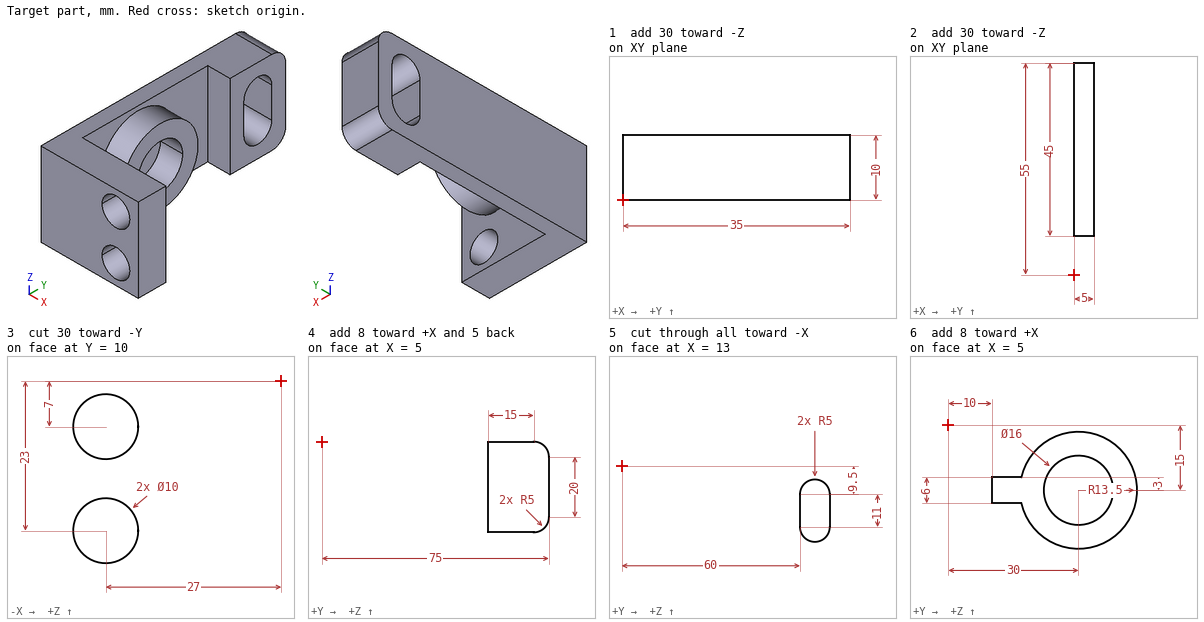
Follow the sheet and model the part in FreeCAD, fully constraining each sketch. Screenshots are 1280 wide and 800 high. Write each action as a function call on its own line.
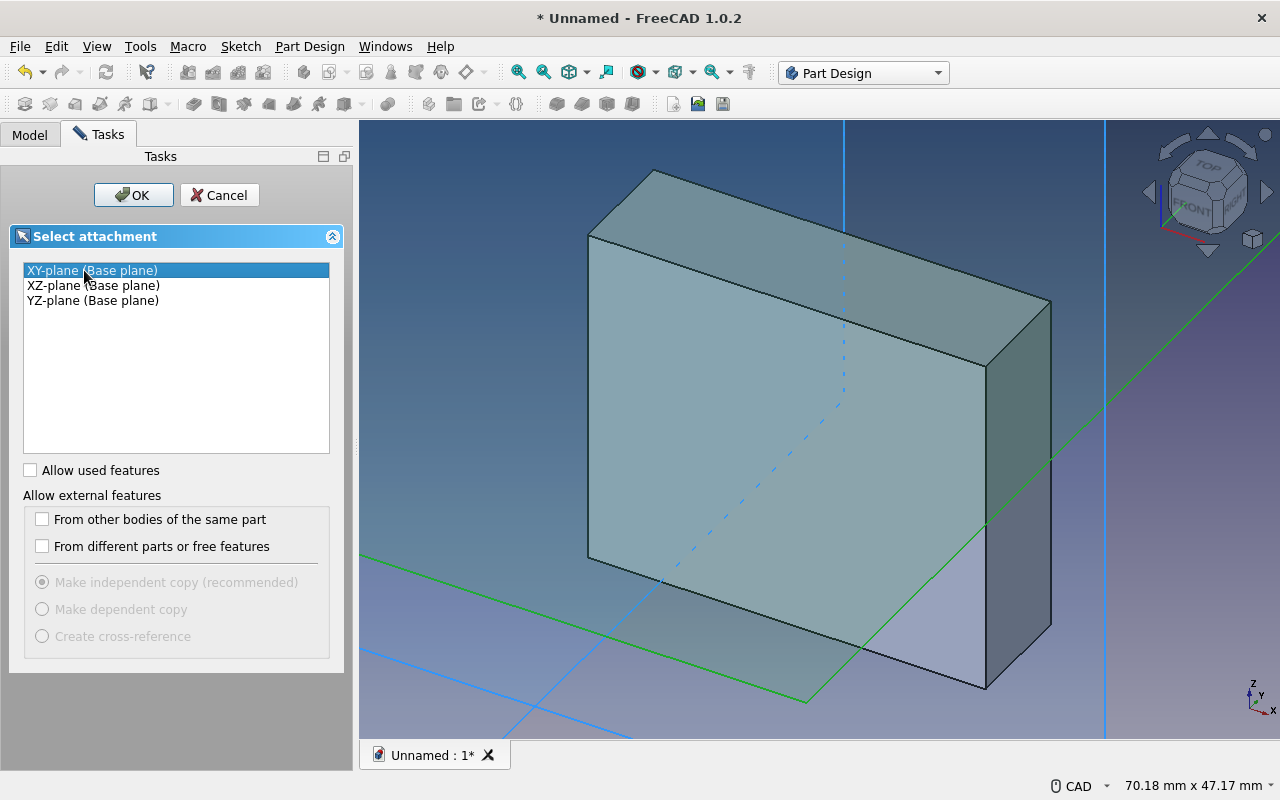
click(134, 195)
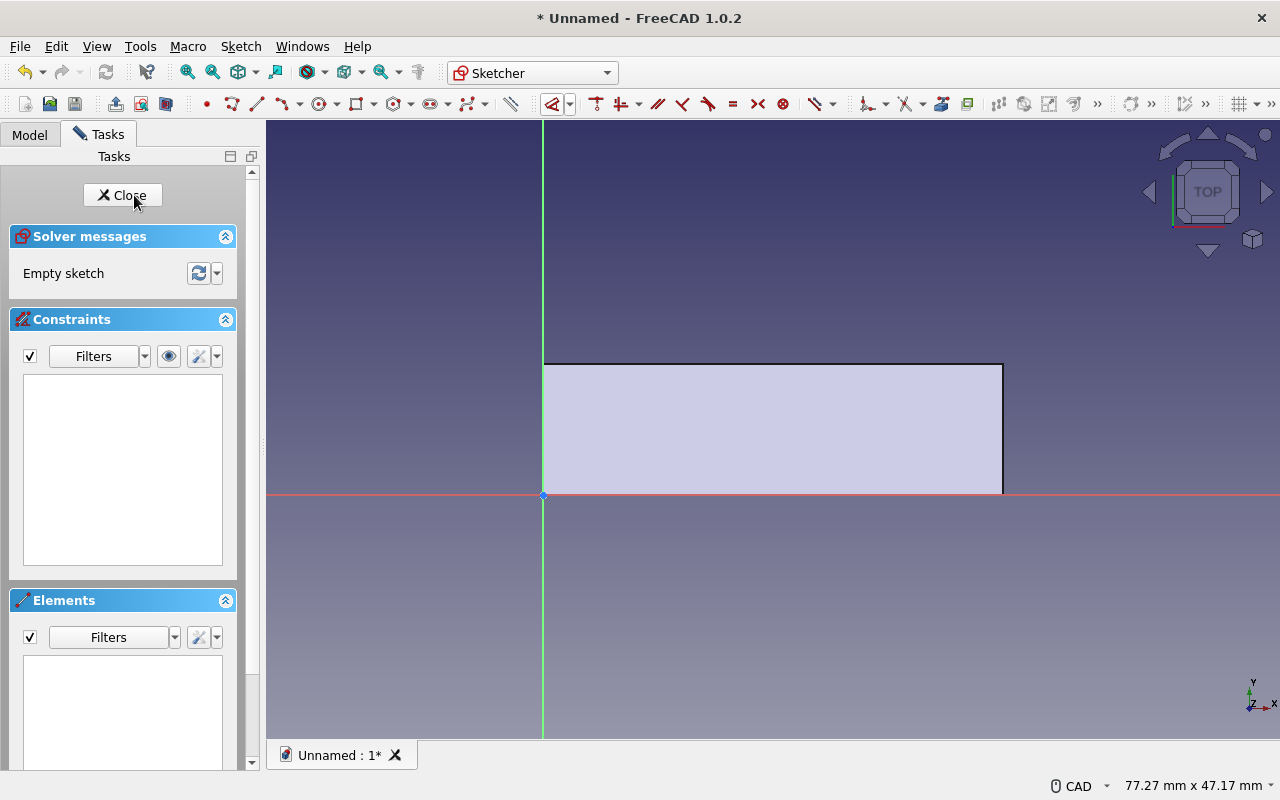
scroll(861, 711, down, 3)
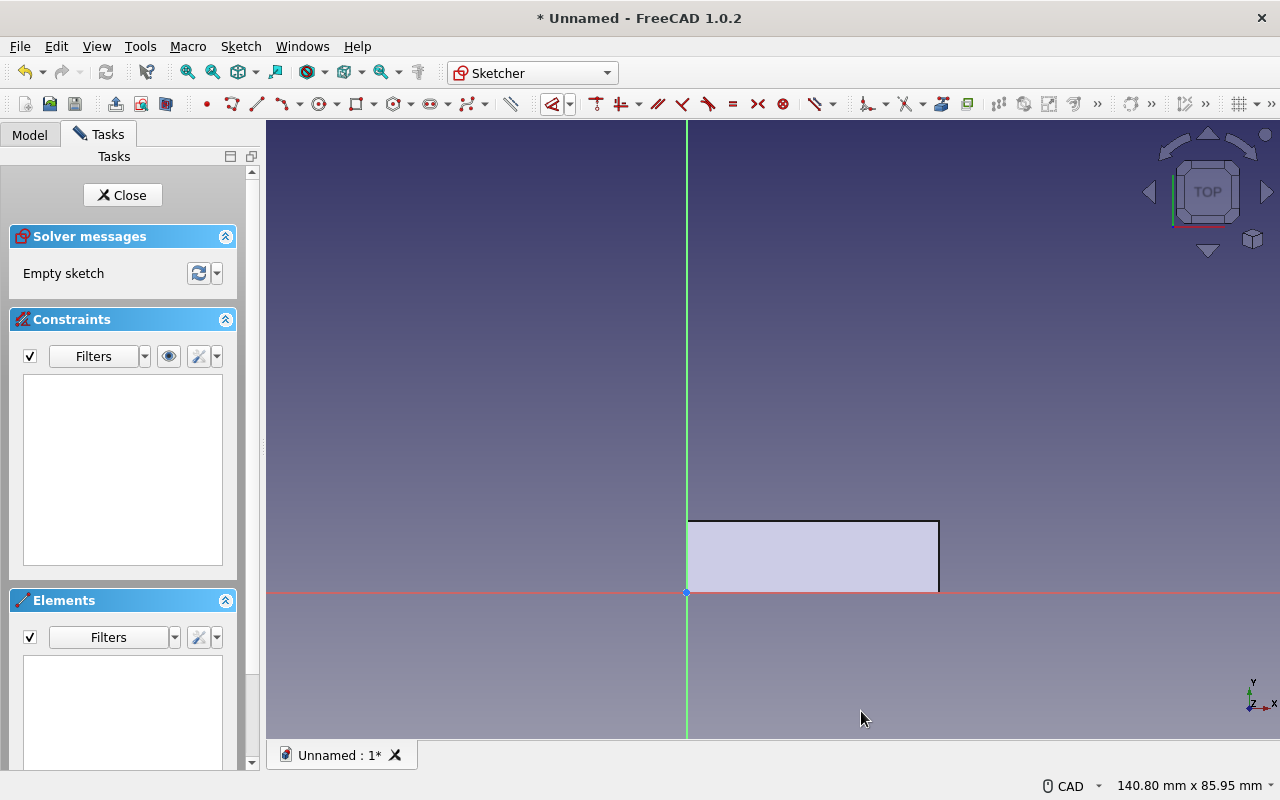
key(g)
key(r)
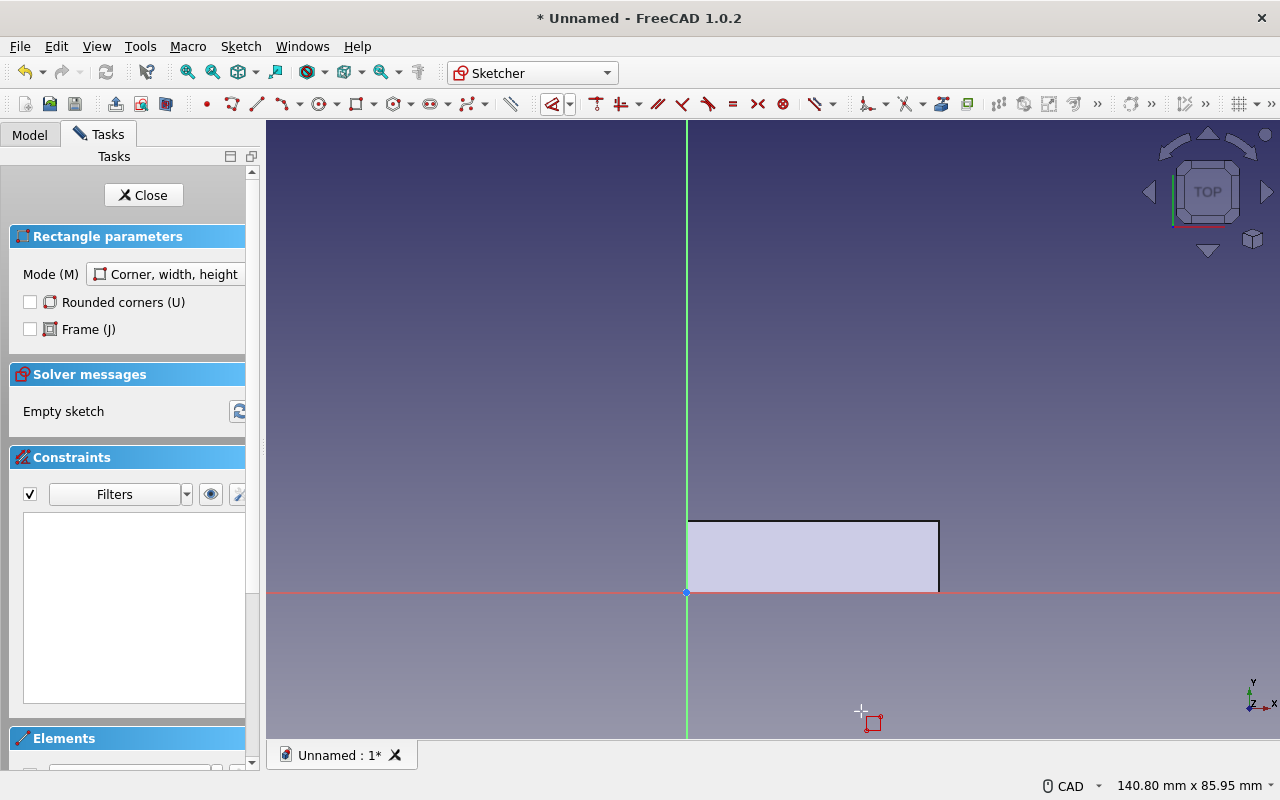
click(687, 197)
click(723, 521)
key(Escape)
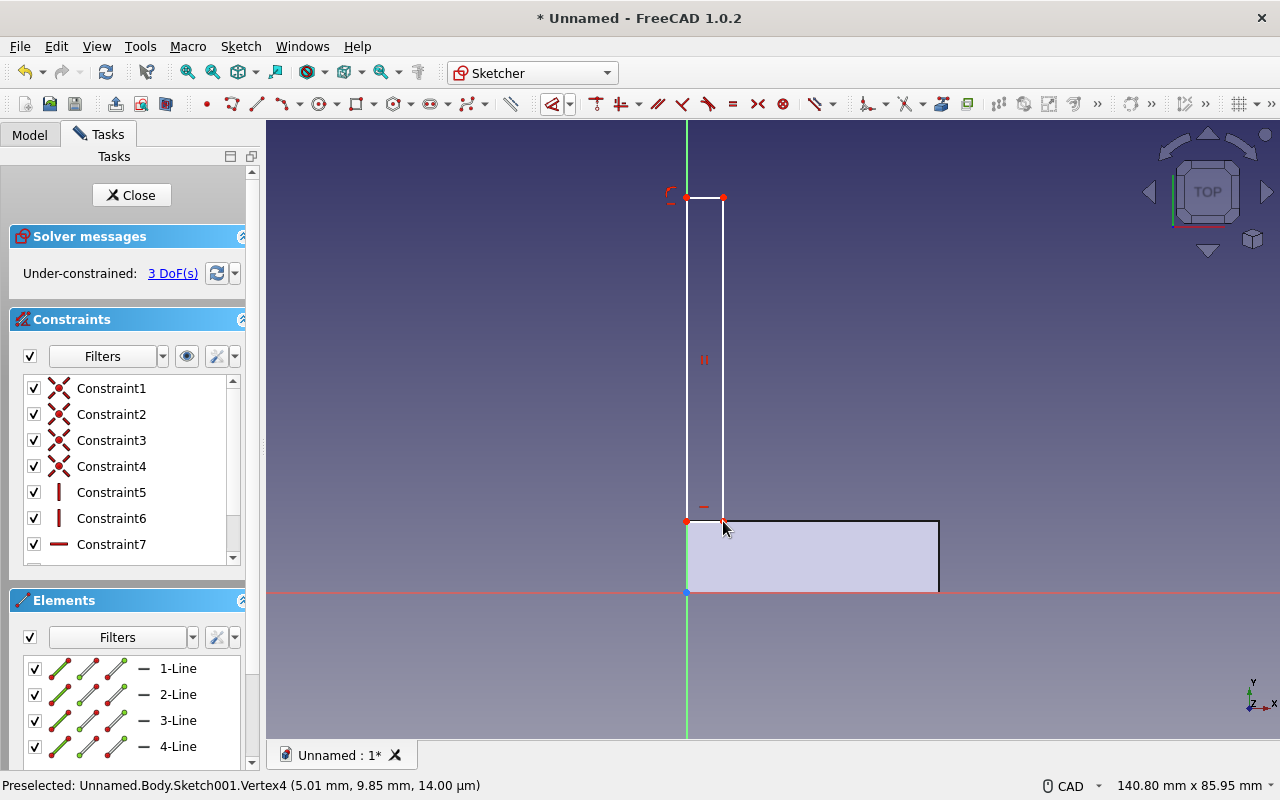
key(d)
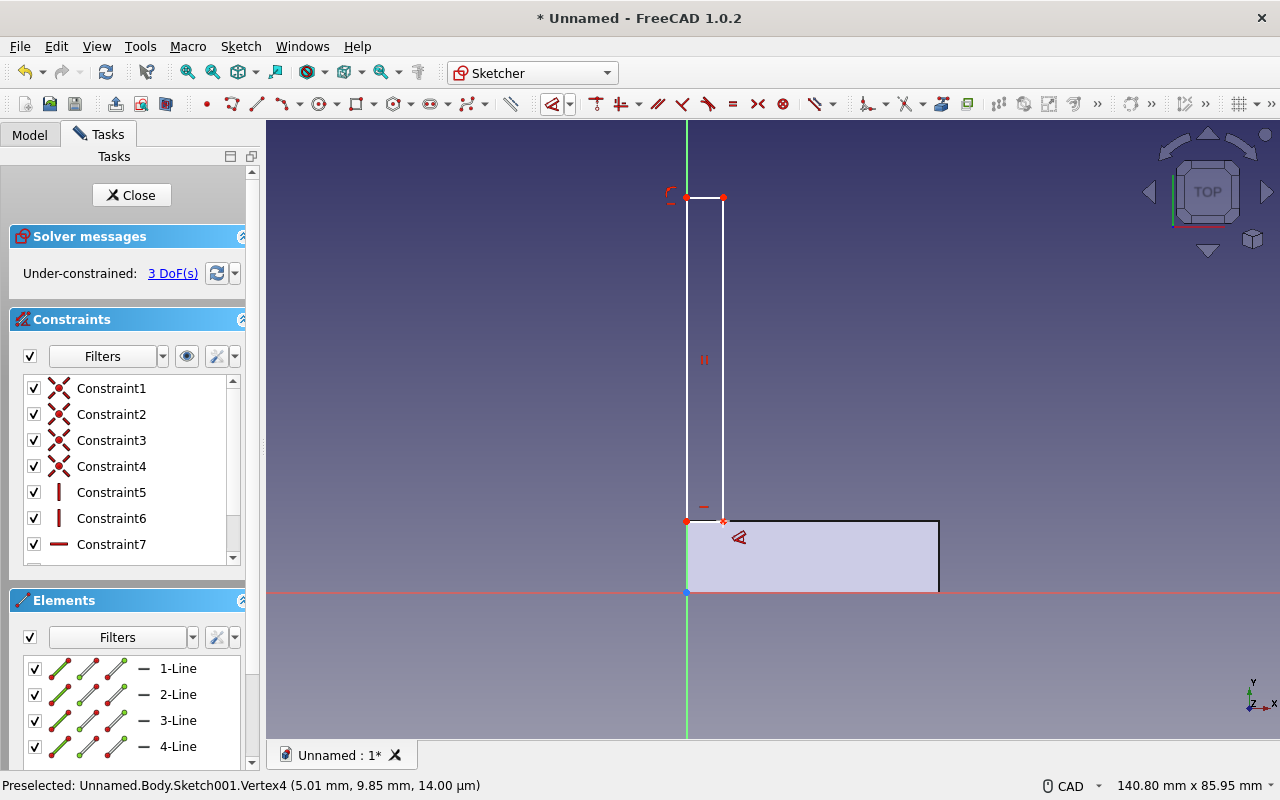
scroll(698, 522, up, 2)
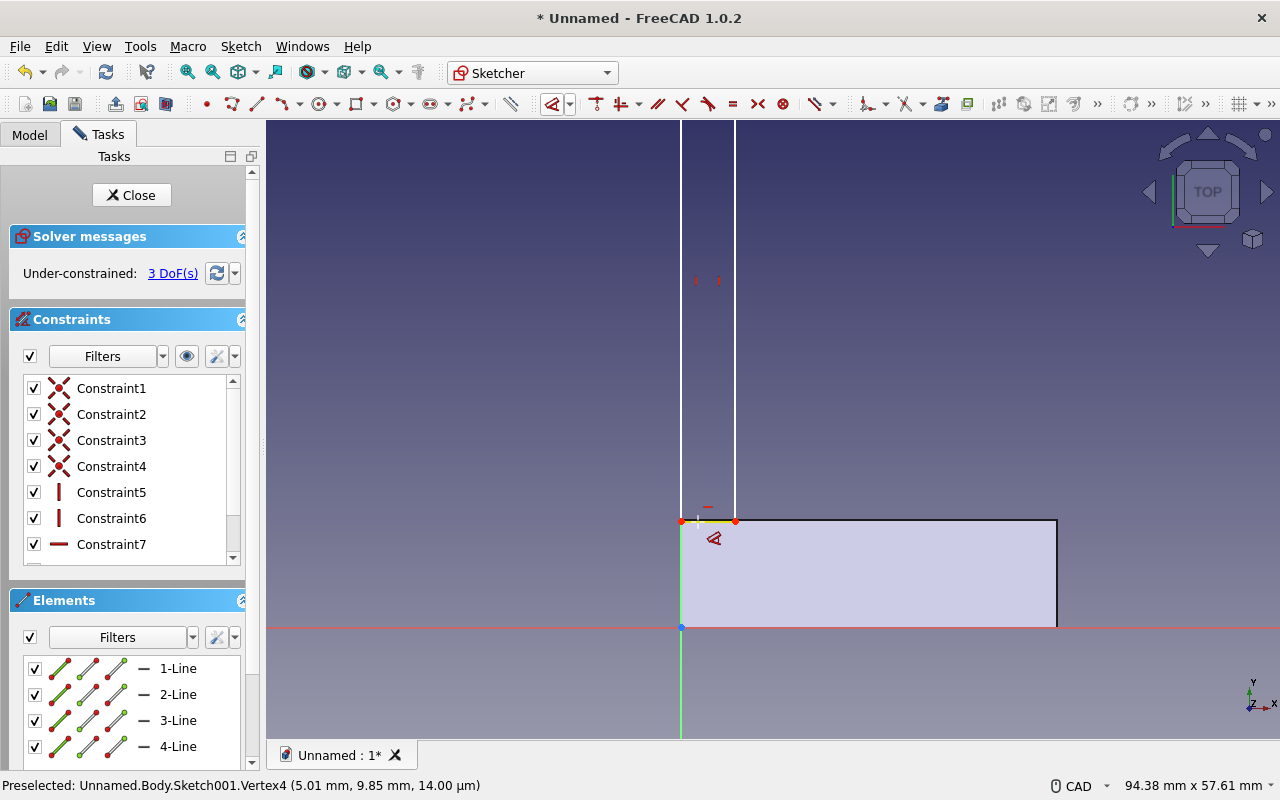
click(697, 522)
click(708, 556)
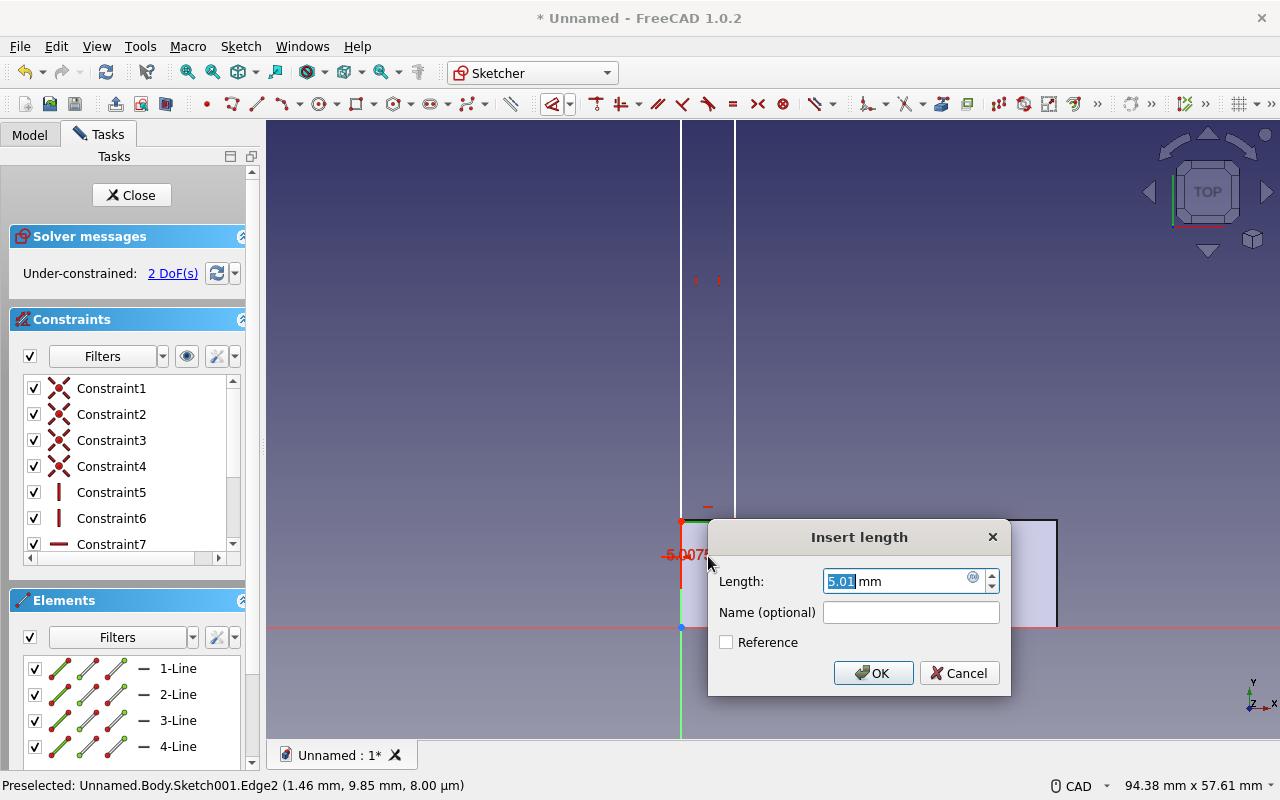
text(5)
key(Return)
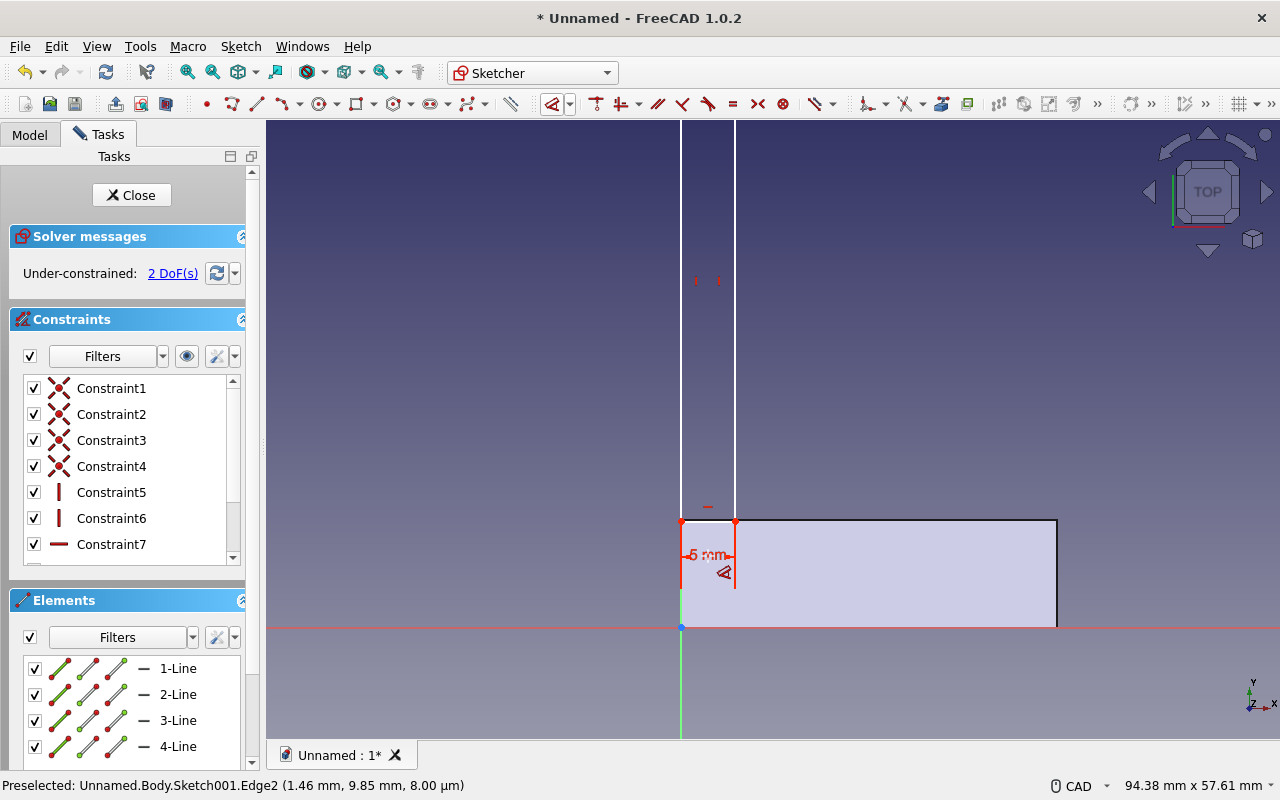
click(681, 183)
click(647, 335)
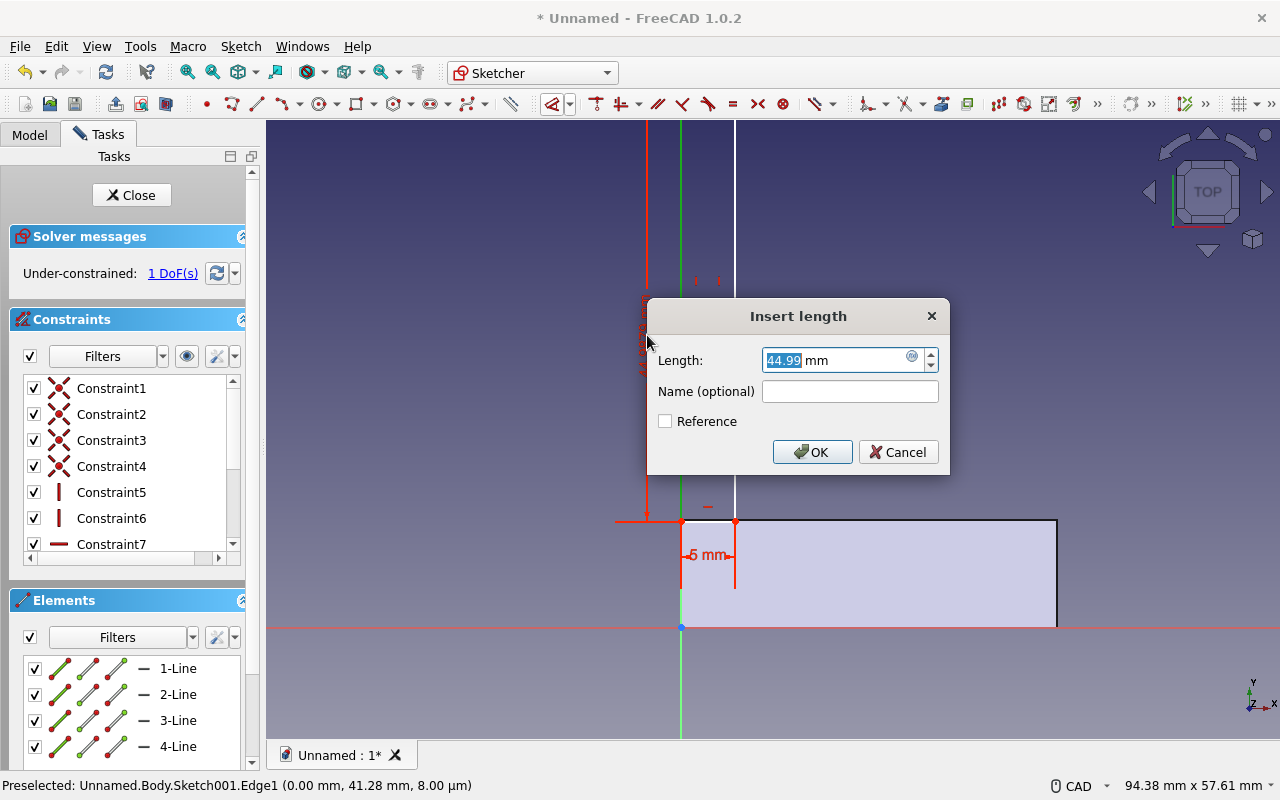
text(45)
key(Return)